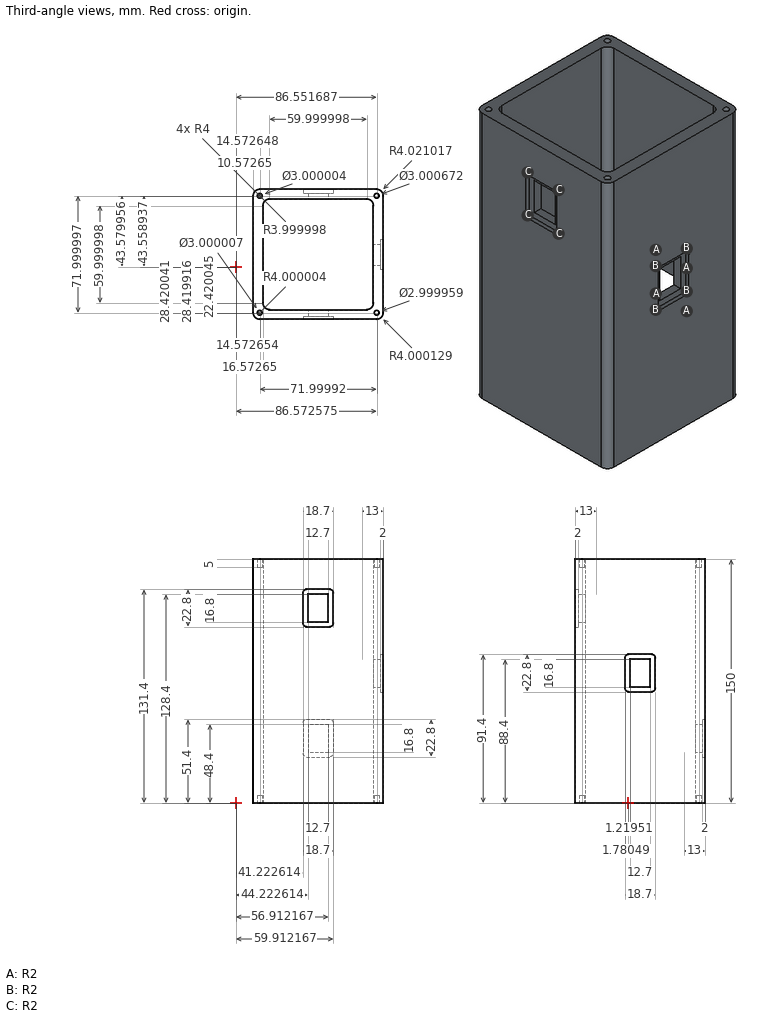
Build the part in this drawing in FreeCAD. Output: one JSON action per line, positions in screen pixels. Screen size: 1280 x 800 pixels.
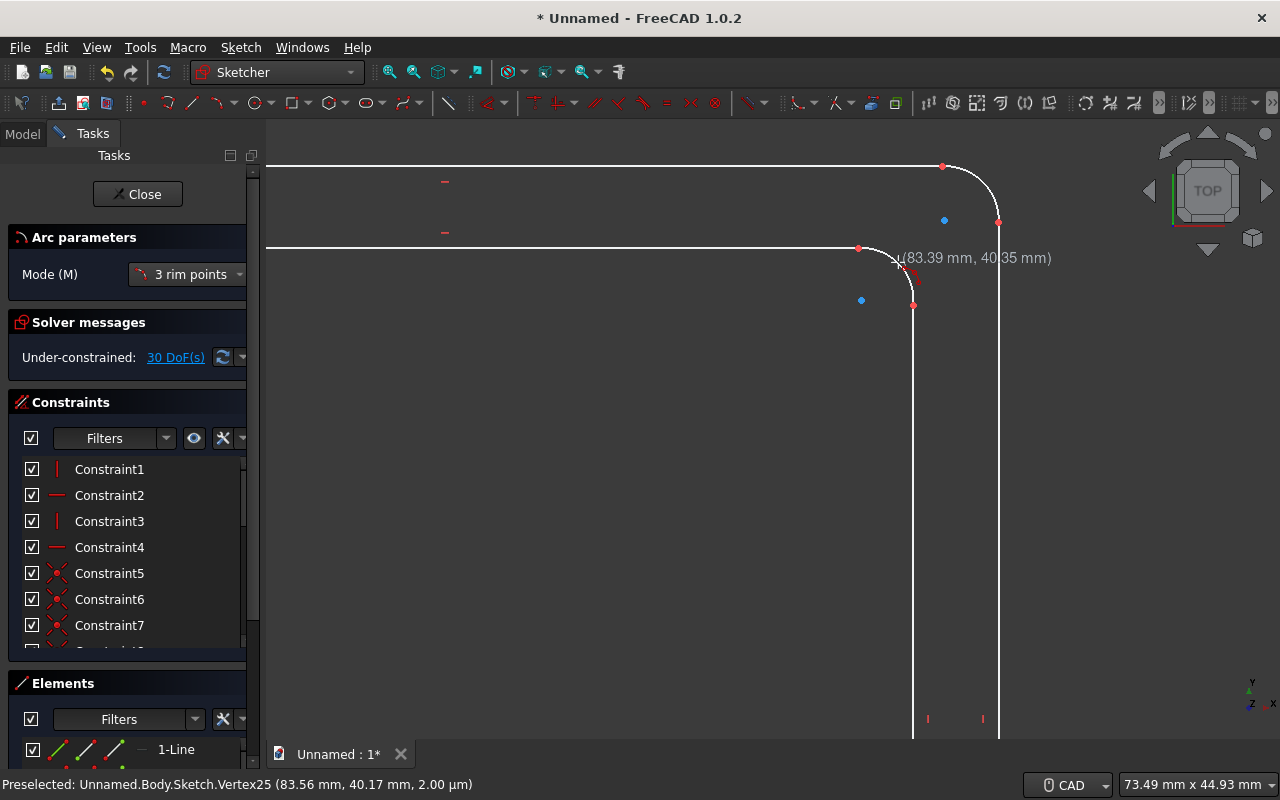
{"action": "scroll", "coordinate": [898, 262], "scroll_direction": "down", "scroll_amount": 5}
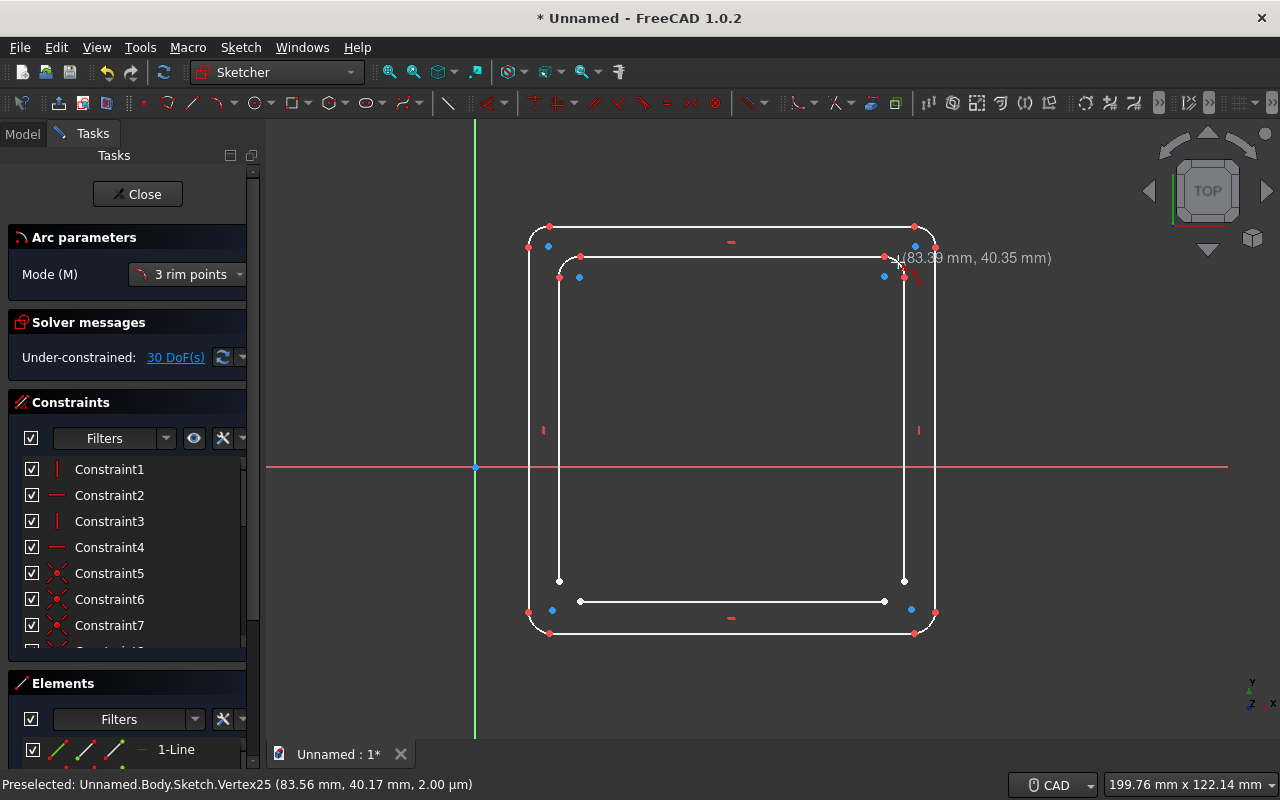
{"action": "left_click", "coordinate": [904, 582]}
{"action": "left_click", "coordinate": [884, 602]}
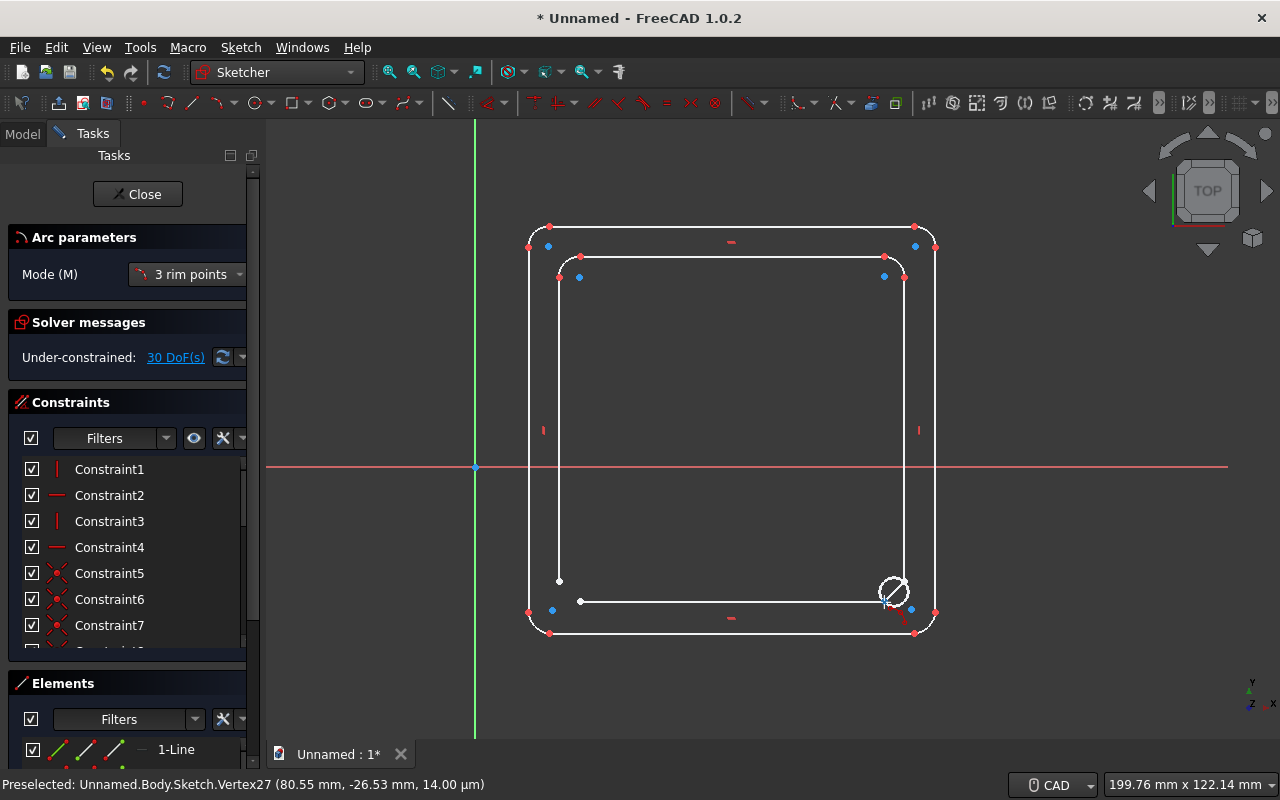
{"action": "scroll", "coordinate": [898, 596], "scroll_direction": "up", "scroll_amount": 5}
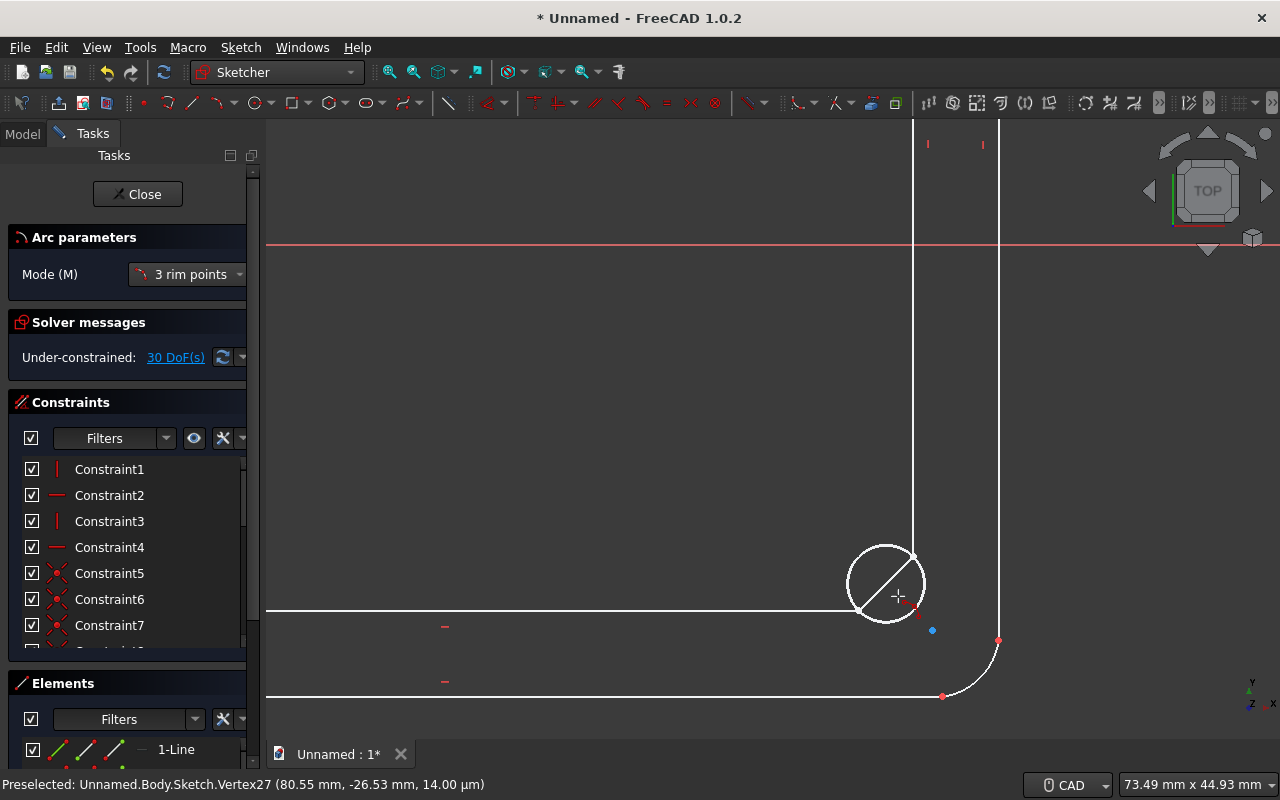
{"action": "left_click", "coordinate": [898, 593]}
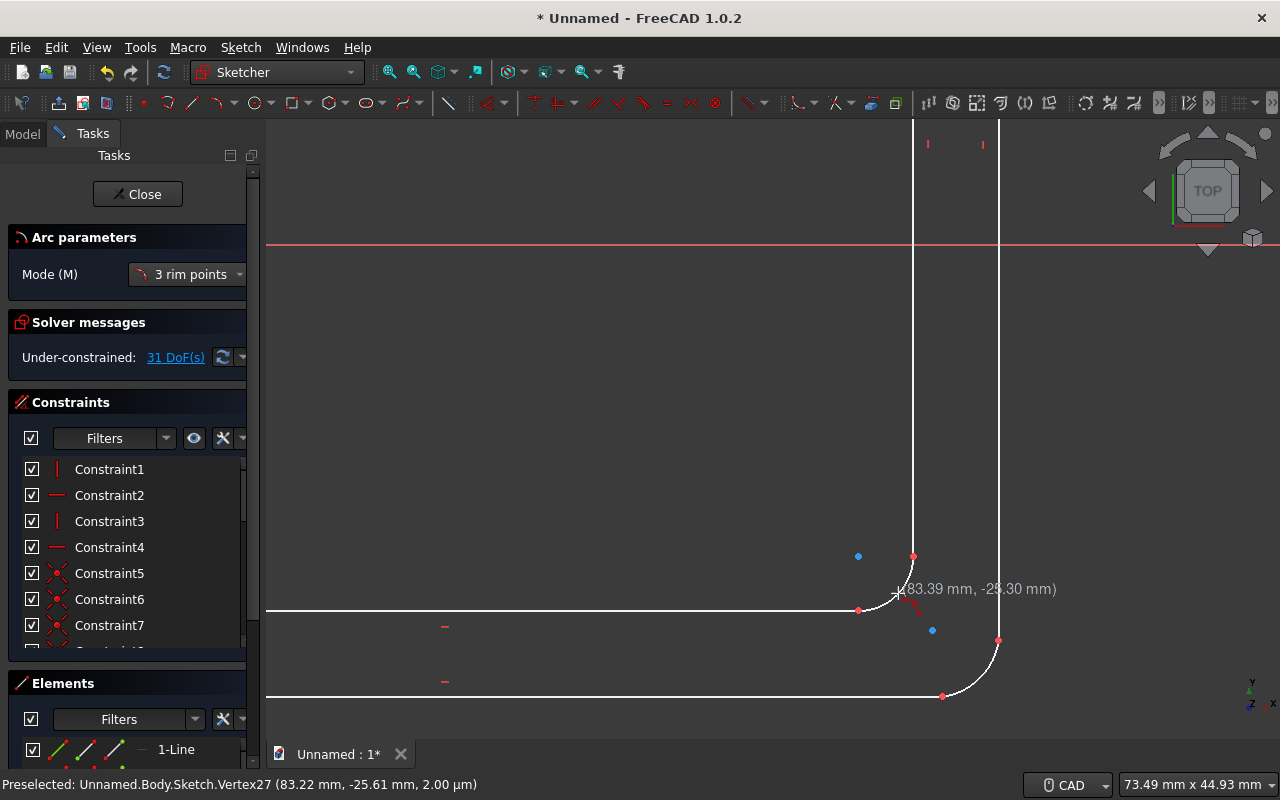
{"action": "scroll", "coordinate": [898, 597], "scroll_direction": "down", "scroll_amount": 5}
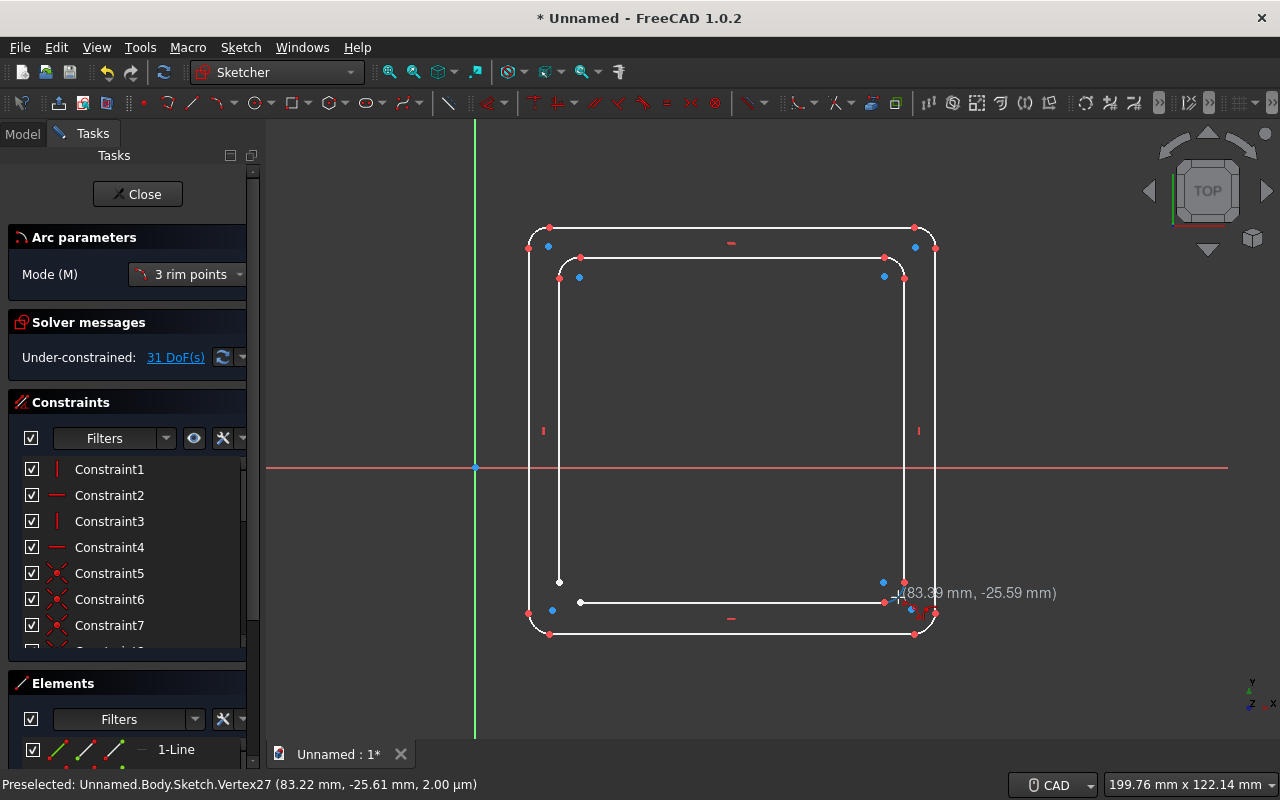
{"action": "left_click", "coordinate": [580, 603]}
{"action": "left_click", "coordinate": [559, 583]}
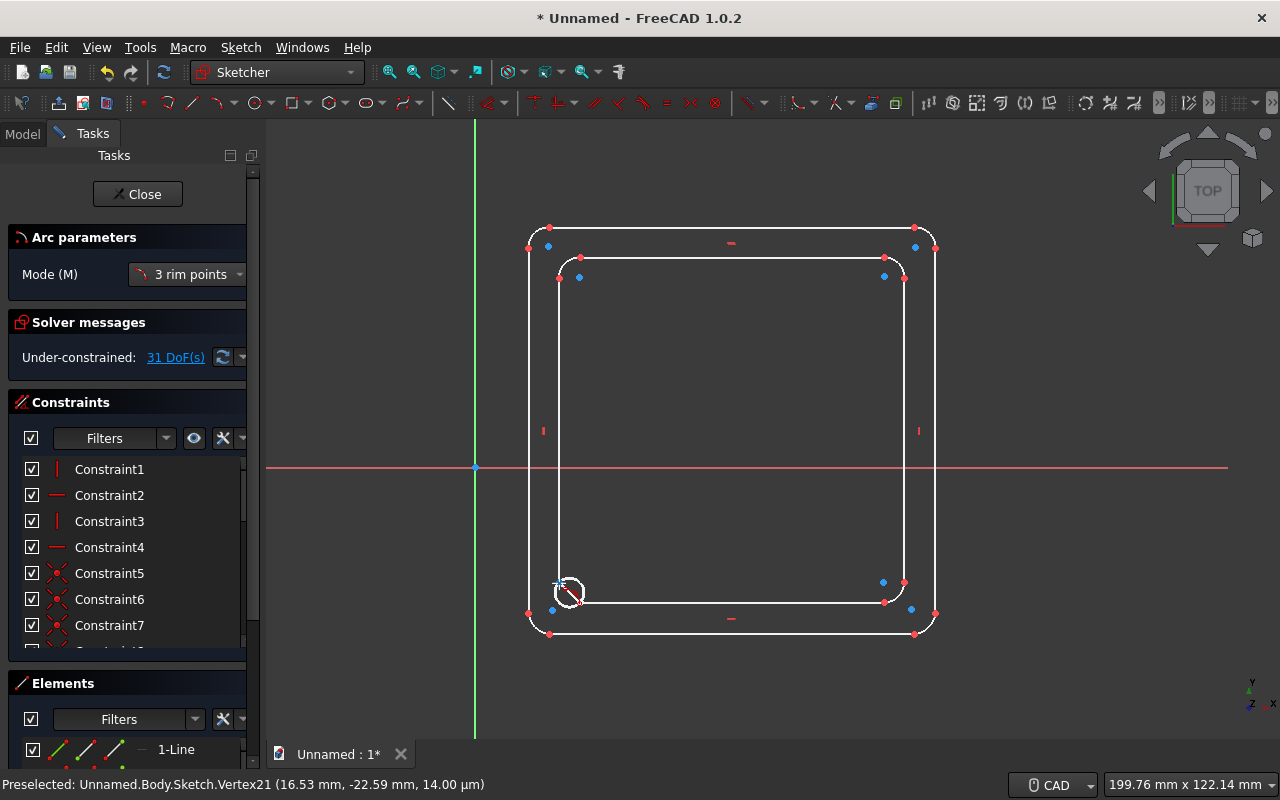
{"action": "scroll", "coordinate": [565, 596], "scroll_direction": "up", "scroll_amount": 5}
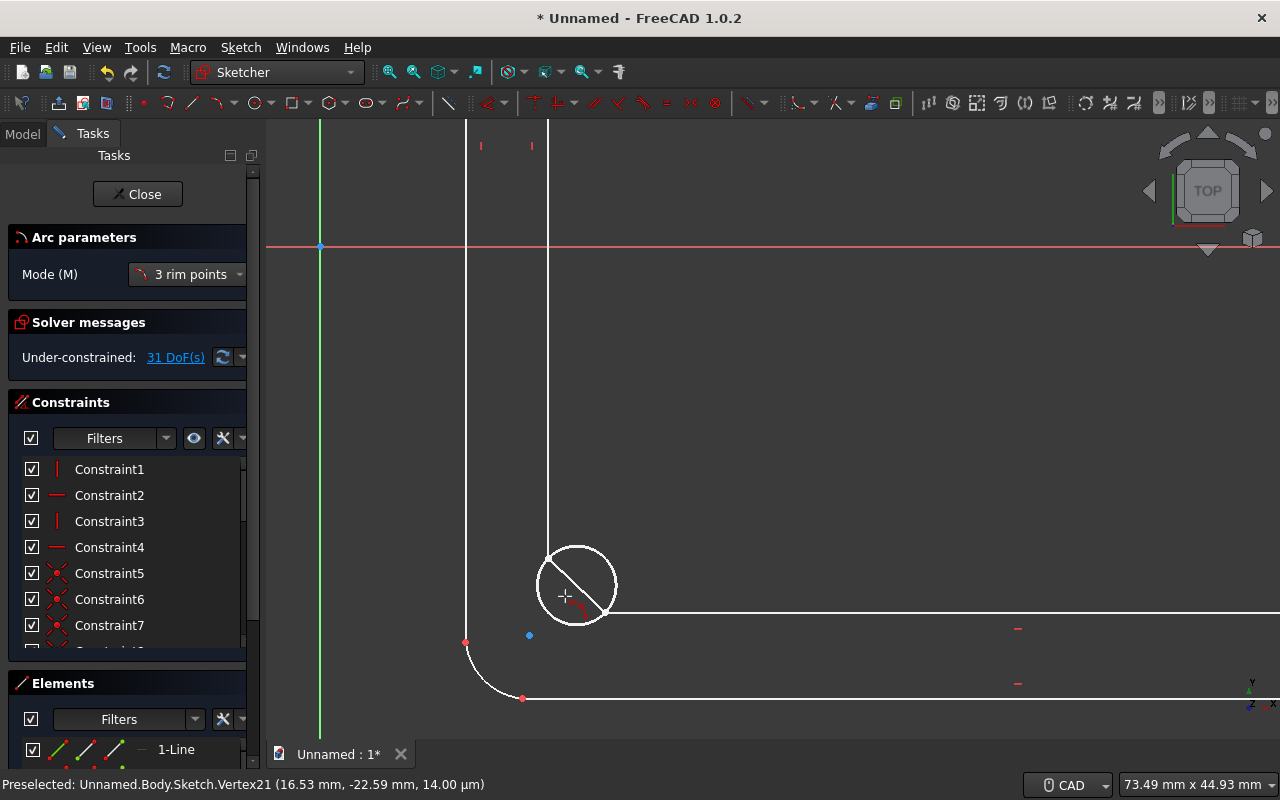
{"action": "left_click", "coordinate": [565, 595]}
{"action": "key", "text": "Escape"}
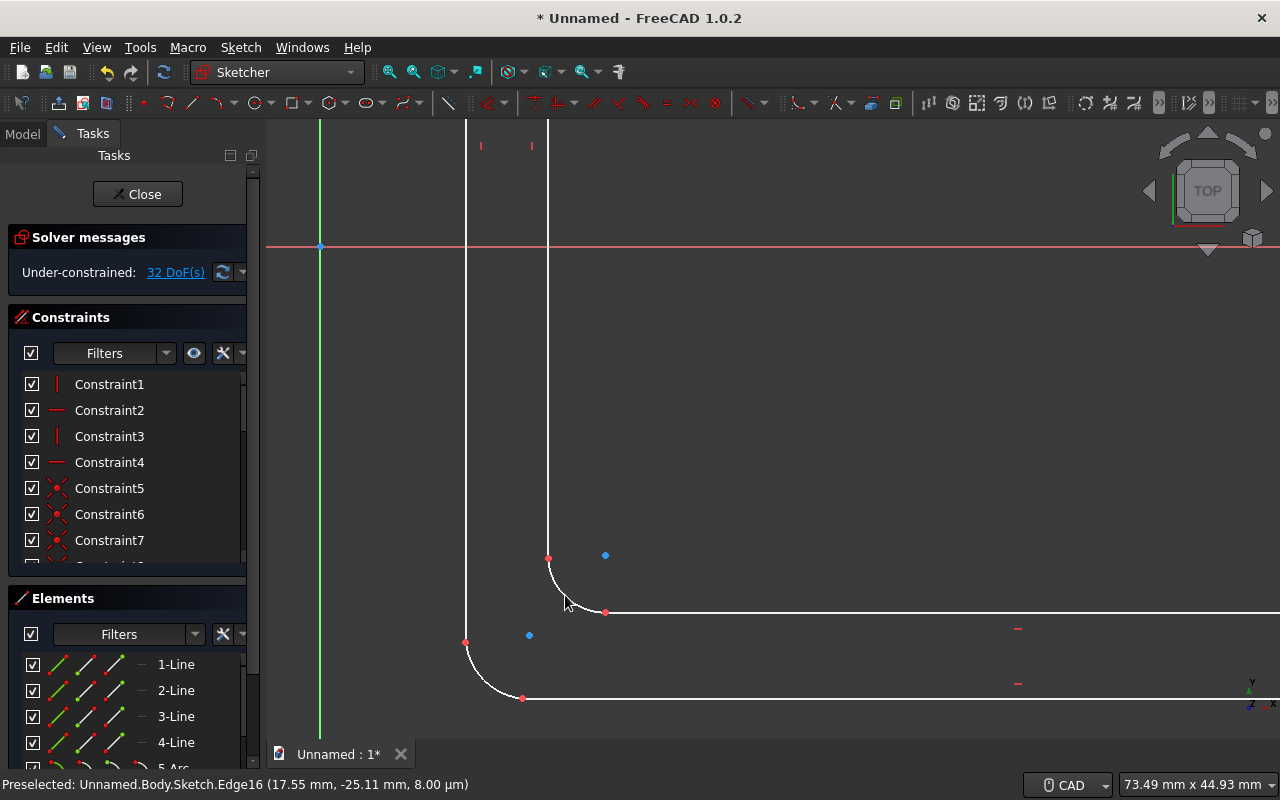
{"action": "left_click", "coordinate": [466, 344]}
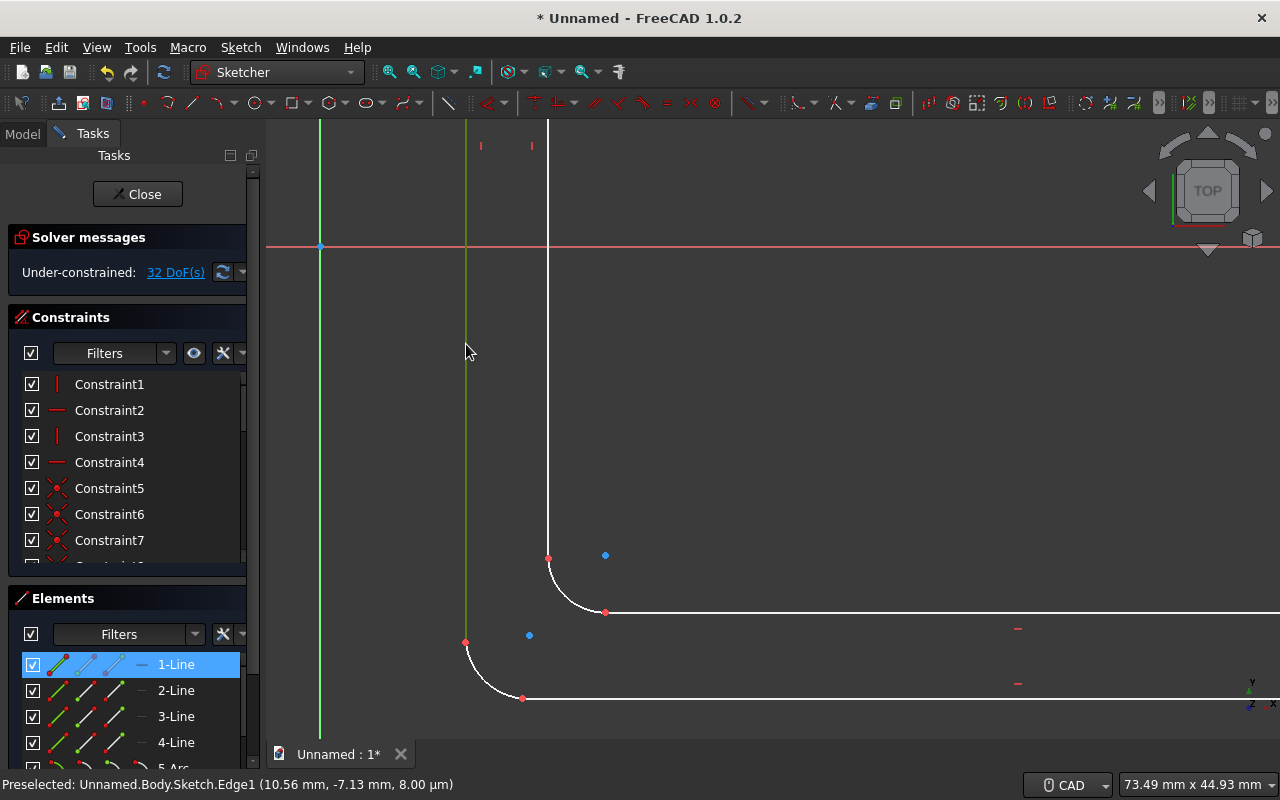
{"action": "left_click", "coordinate": [474, 667]}